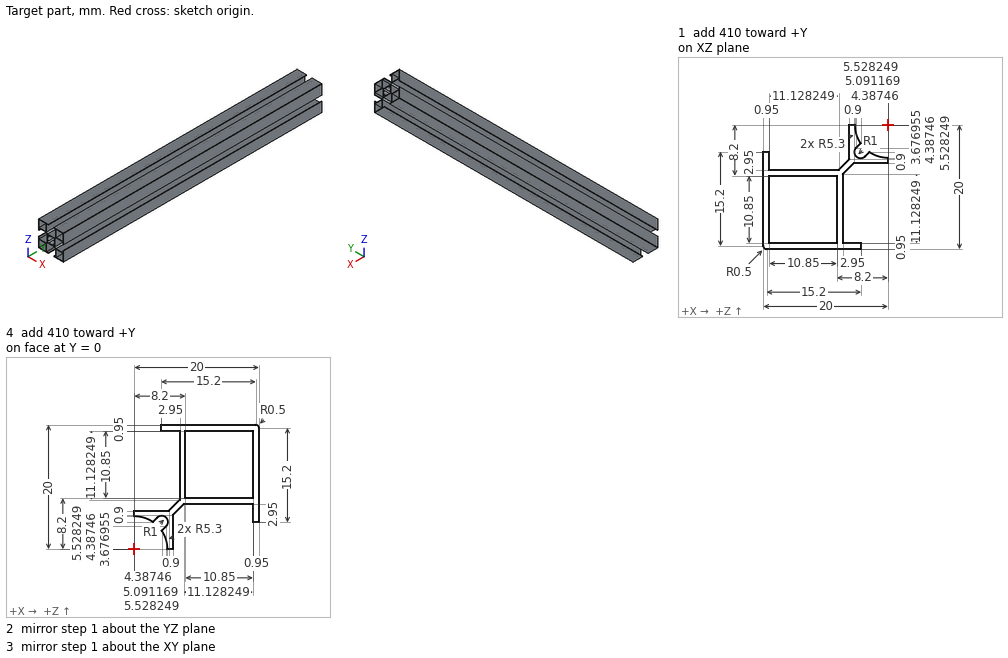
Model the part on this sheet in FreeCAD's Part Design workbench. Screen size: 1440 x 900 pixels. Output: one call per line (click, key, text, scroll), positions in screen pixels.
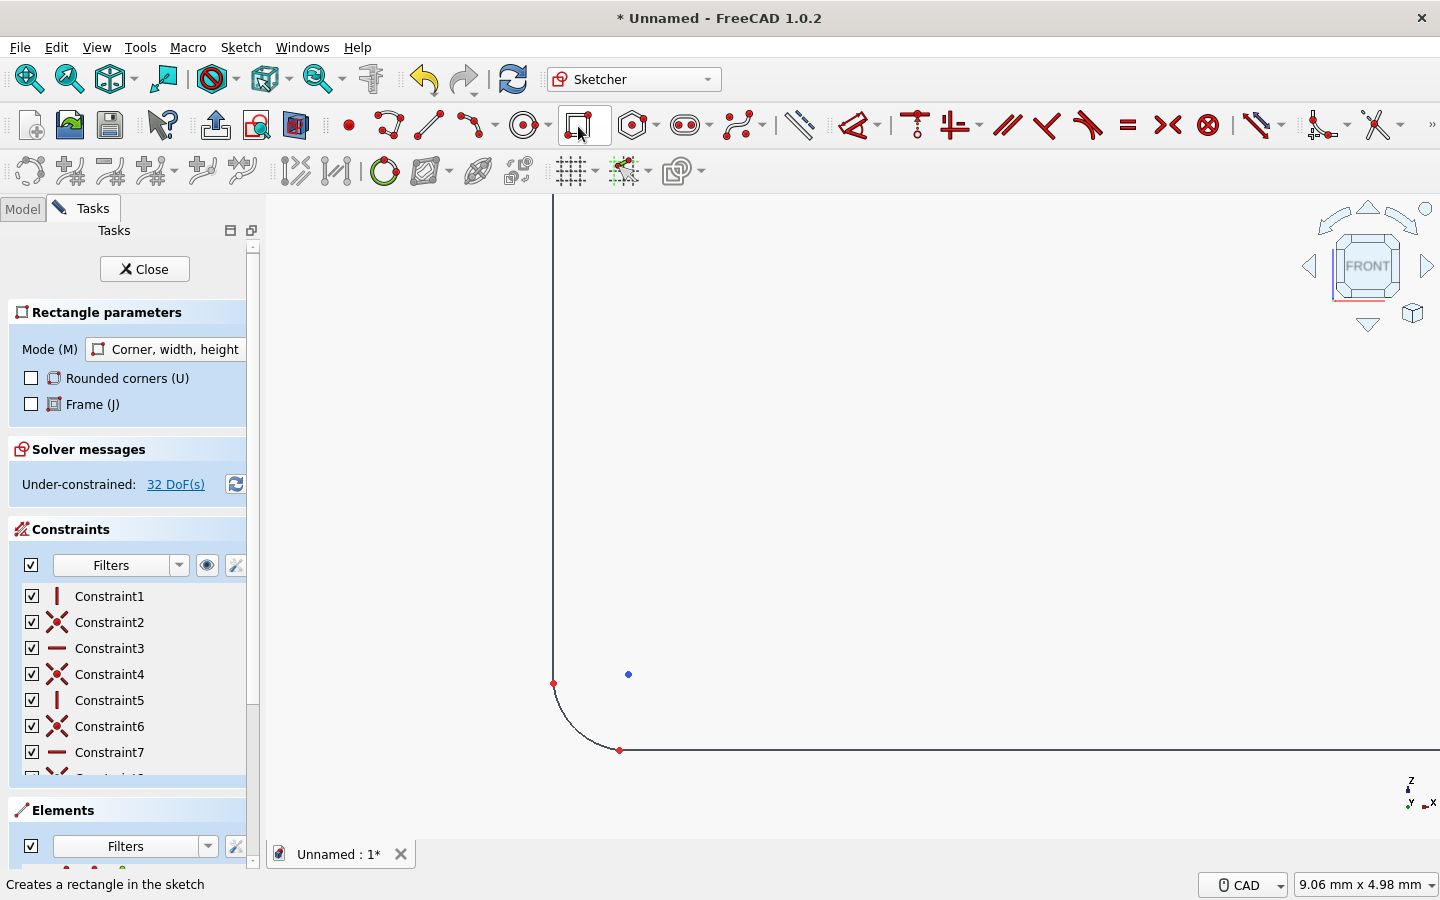
scroll(574, 728, down, 9)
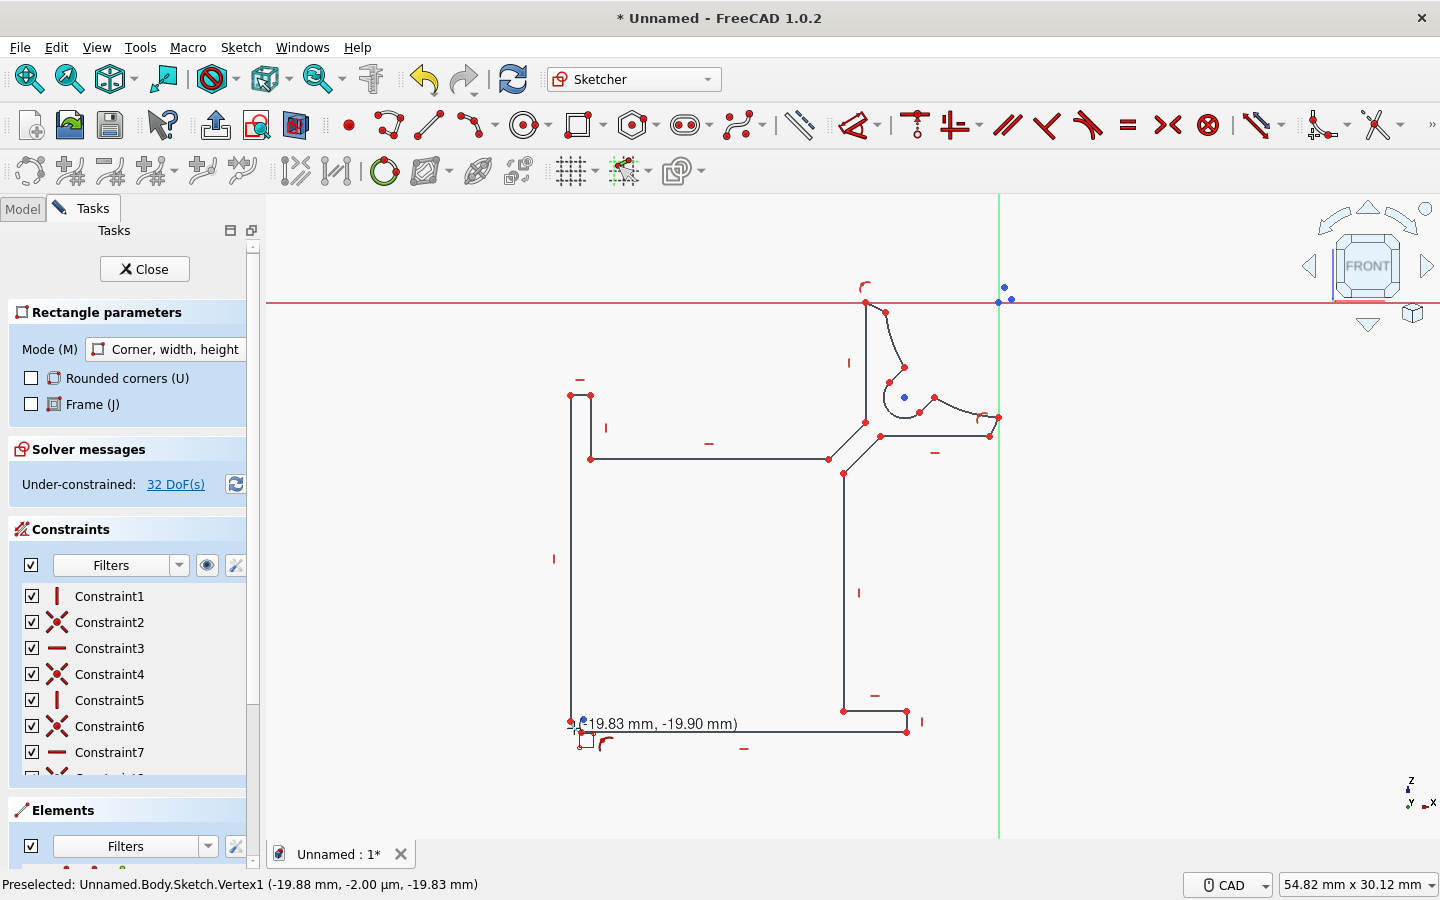
click(591, 478)
click(823, 711)
key(Escape)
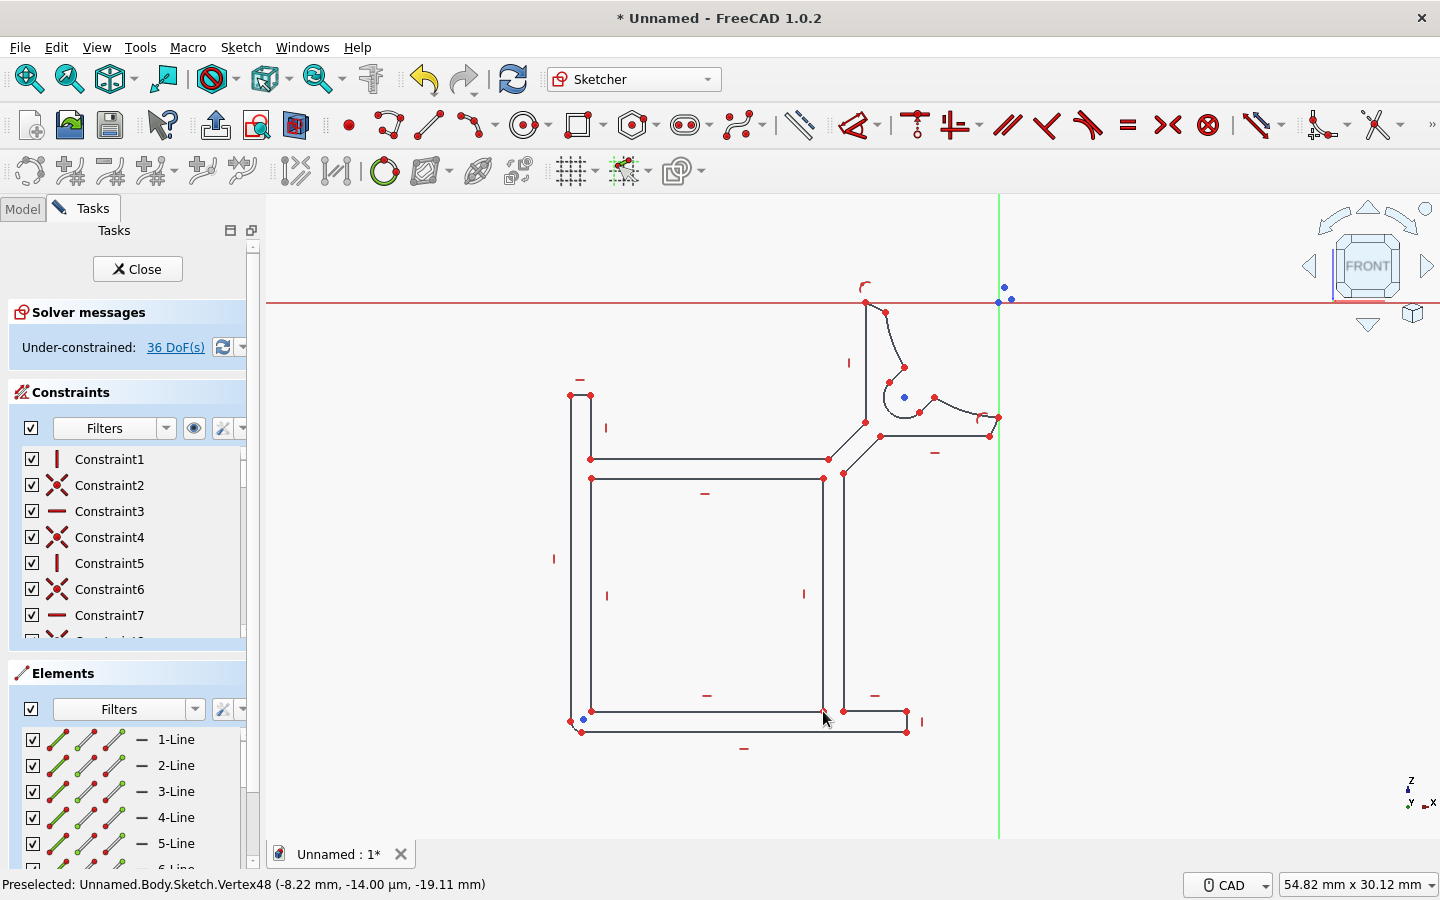
click(571, 624)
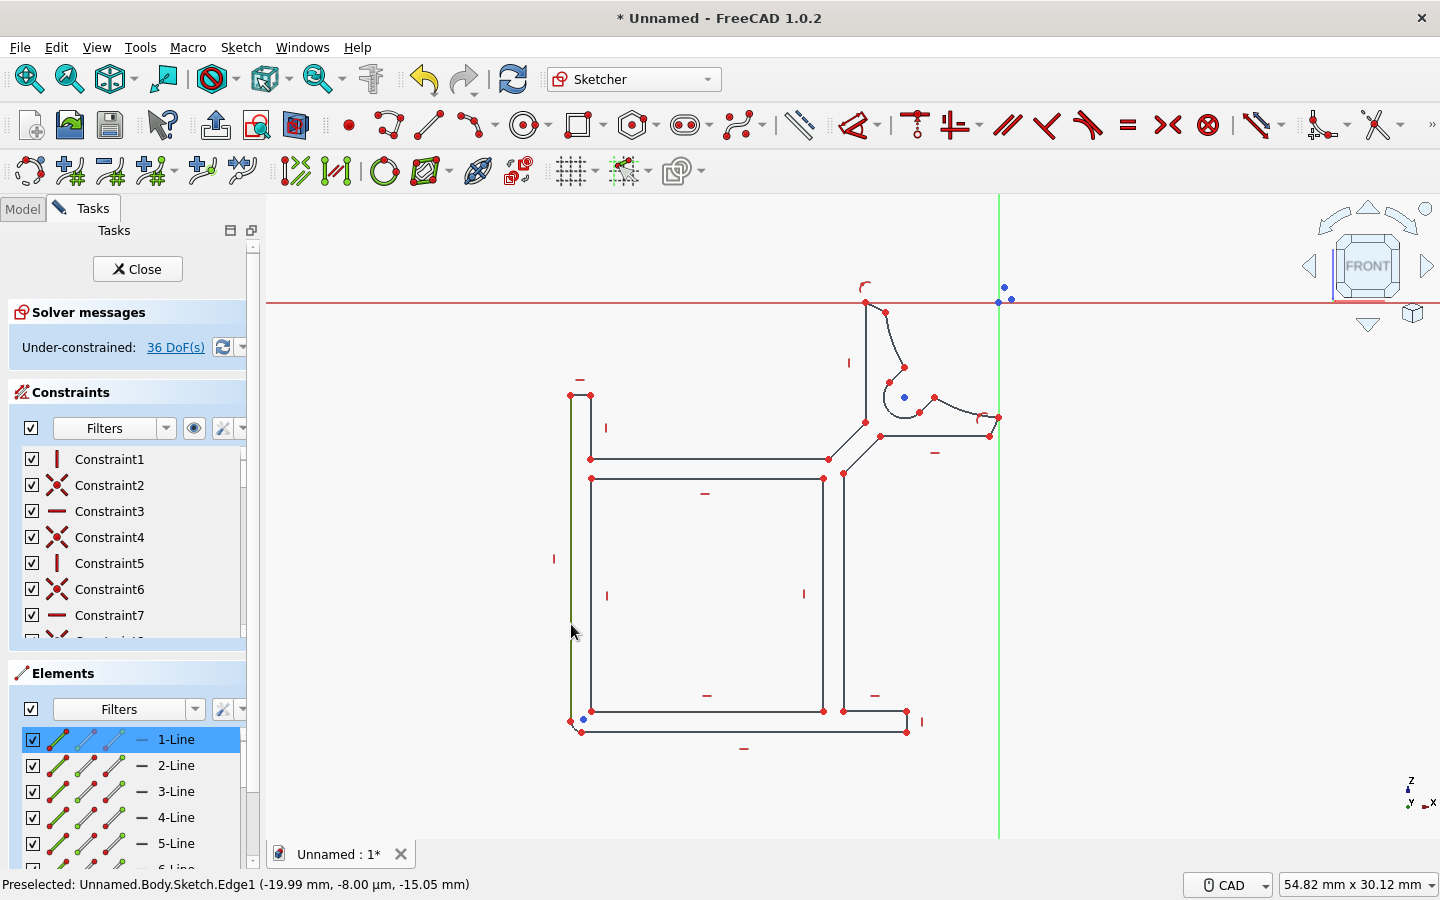
scroll(574, 729, up, 3)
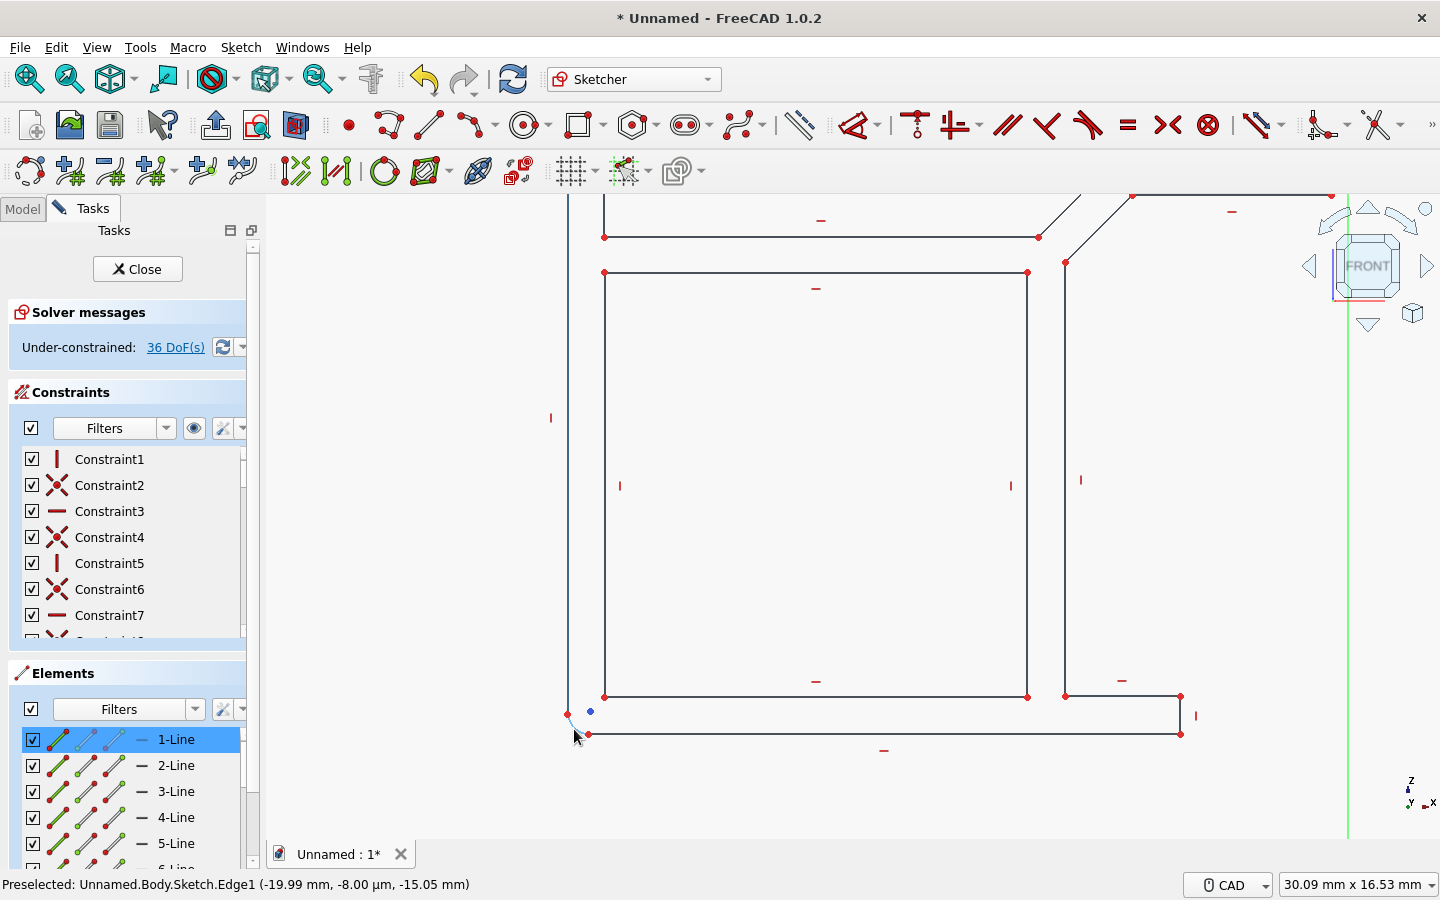
click(575, 728)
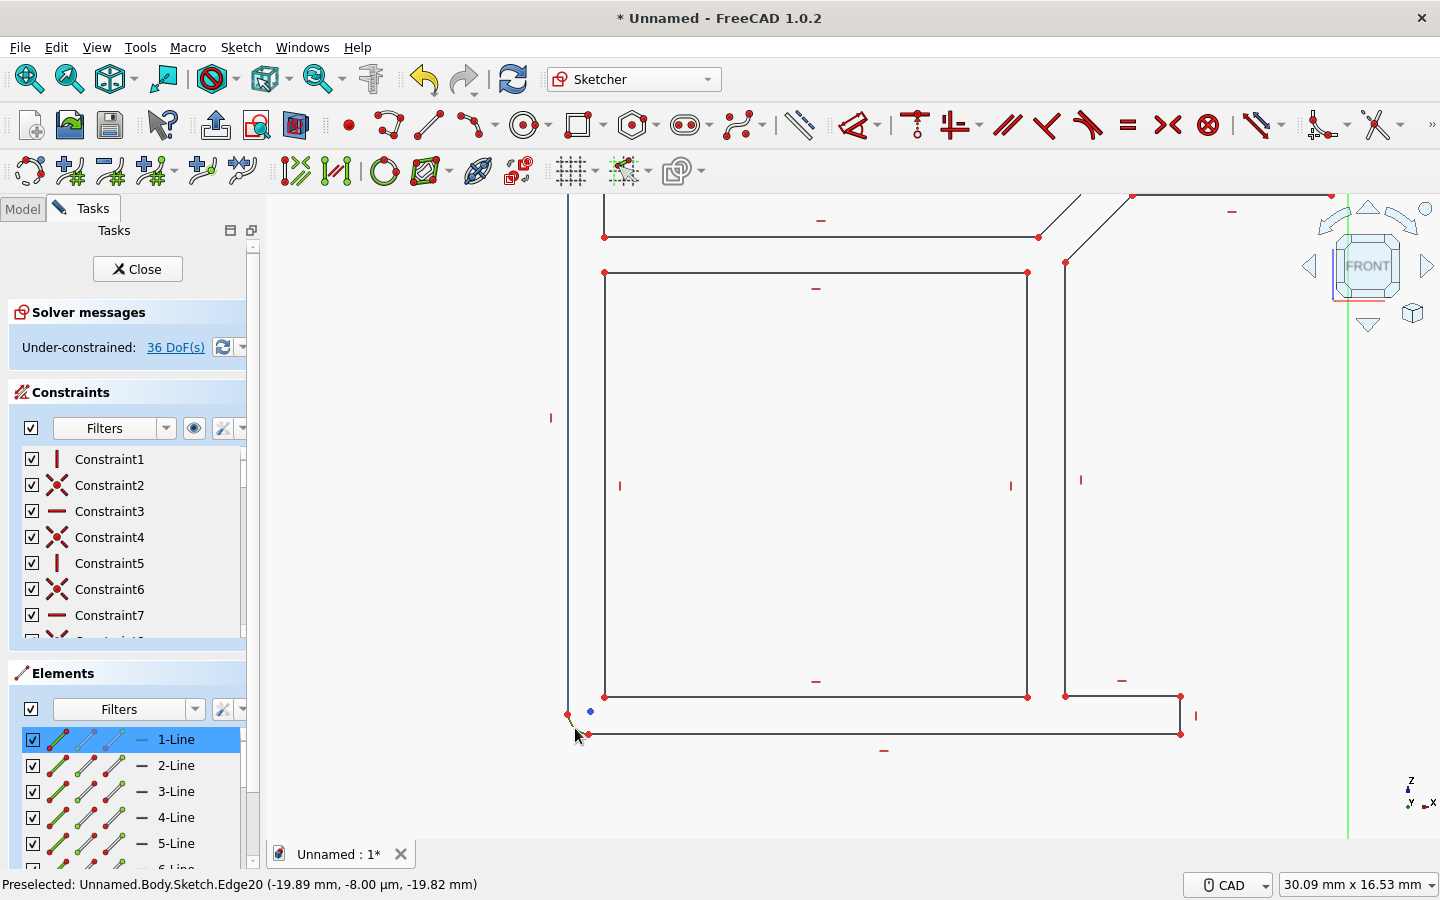
click(1088, 126)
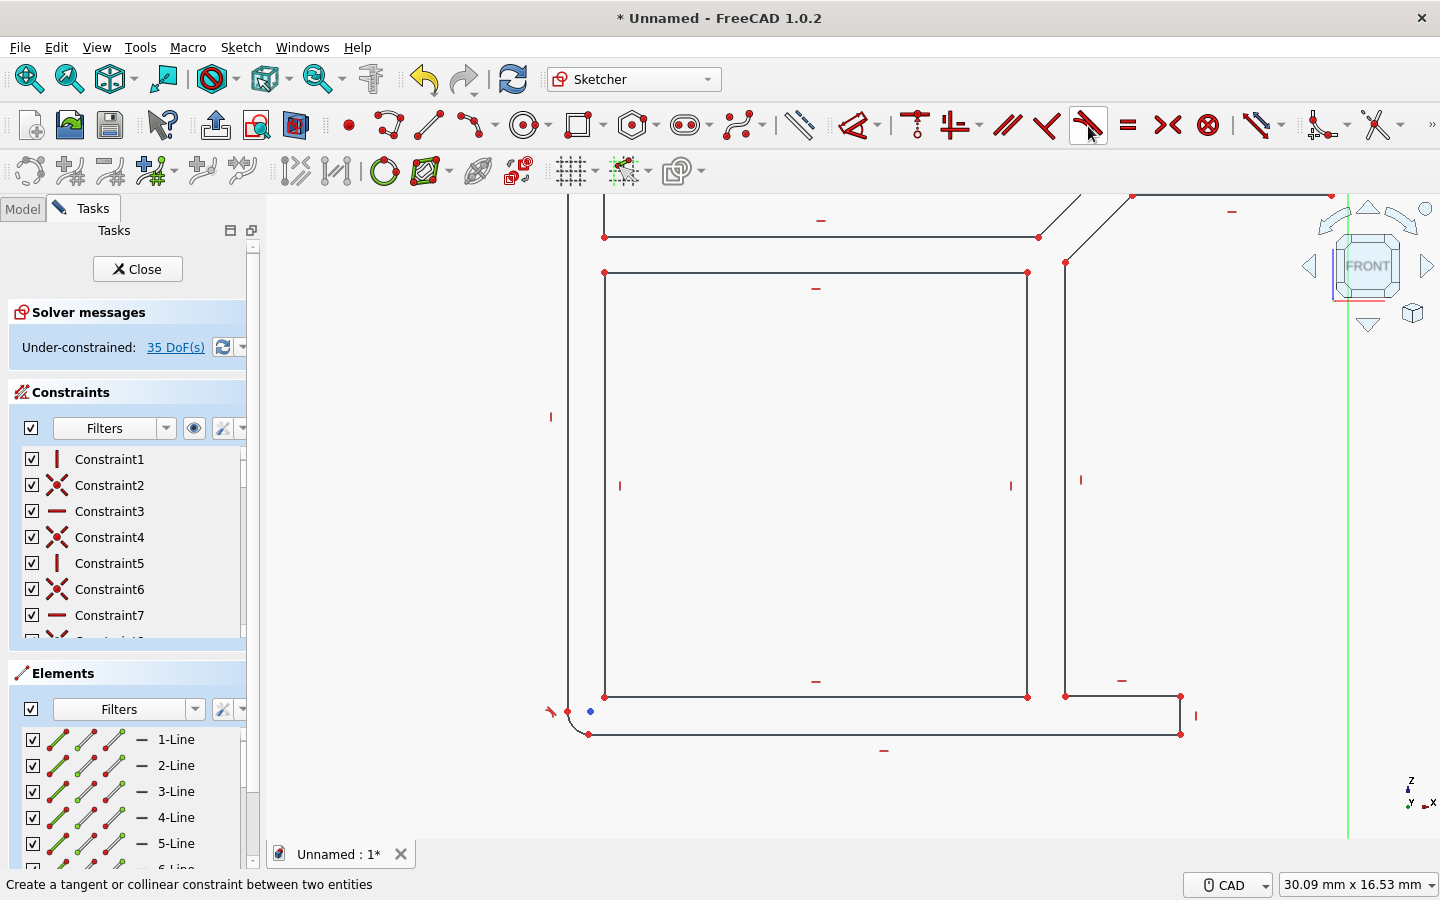
scroll(574, 729, down, 3)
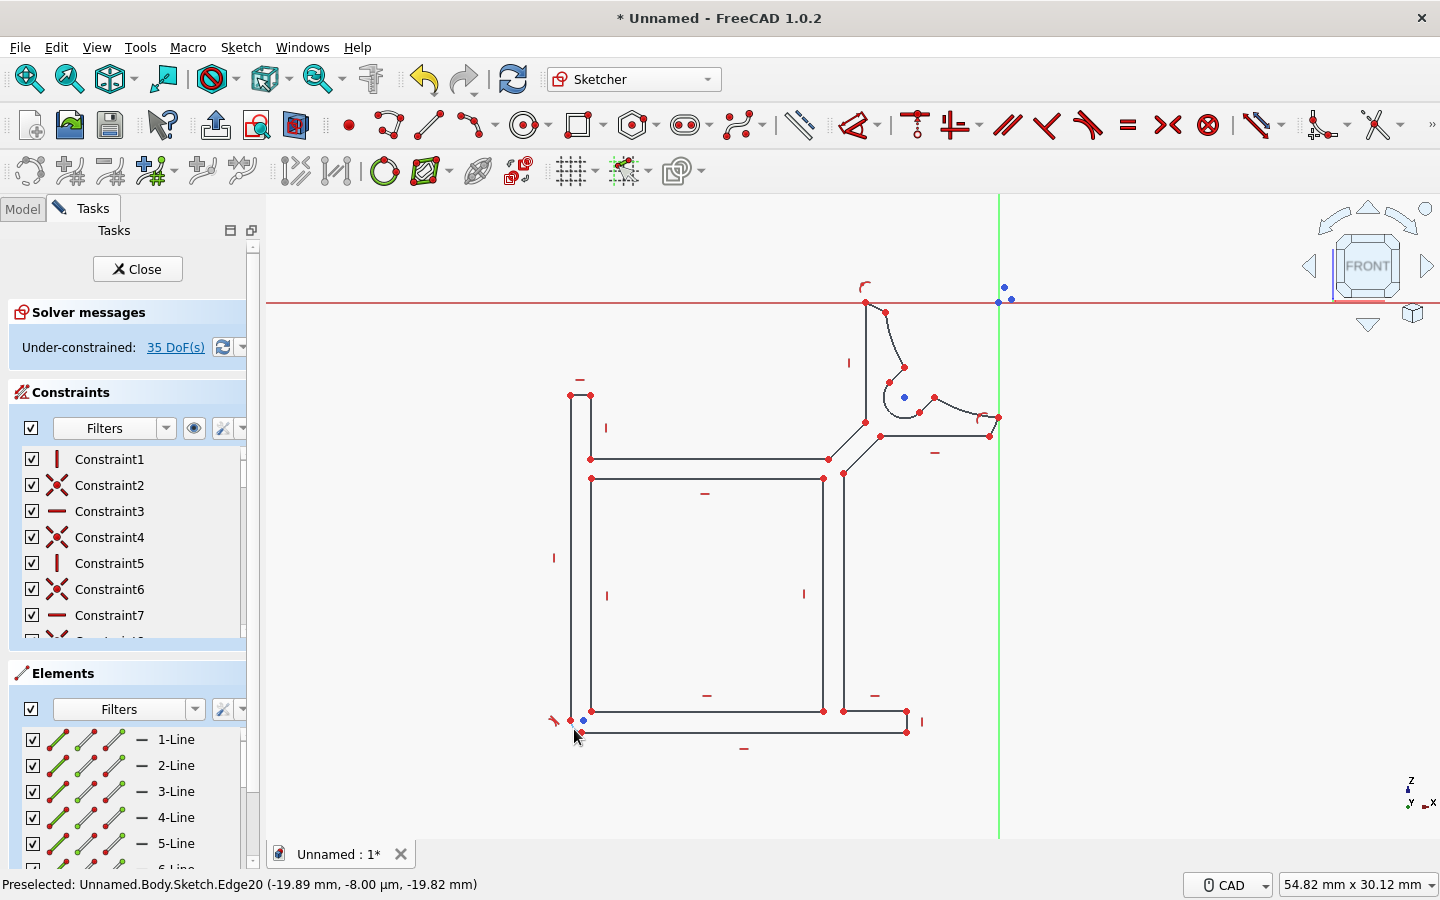
scroll(900, 372, up, 4)